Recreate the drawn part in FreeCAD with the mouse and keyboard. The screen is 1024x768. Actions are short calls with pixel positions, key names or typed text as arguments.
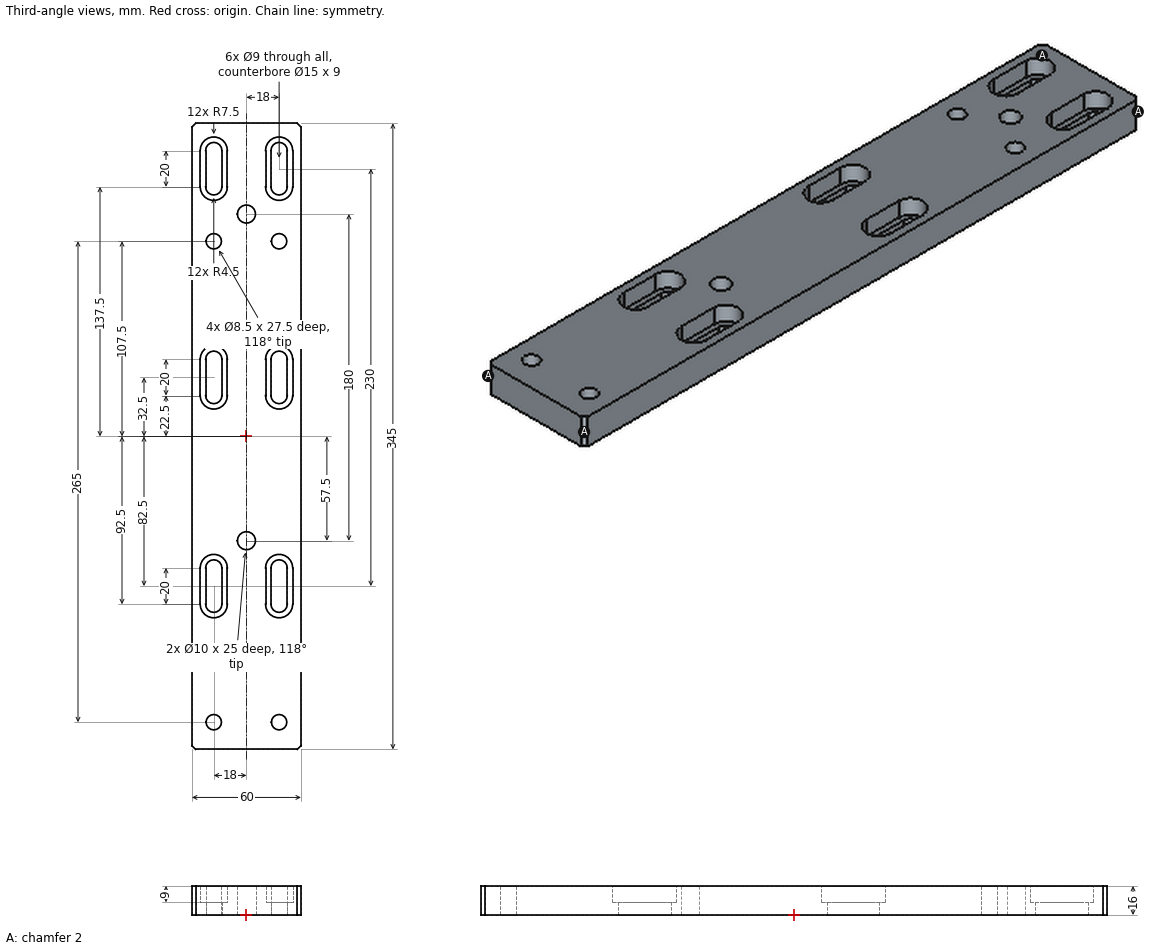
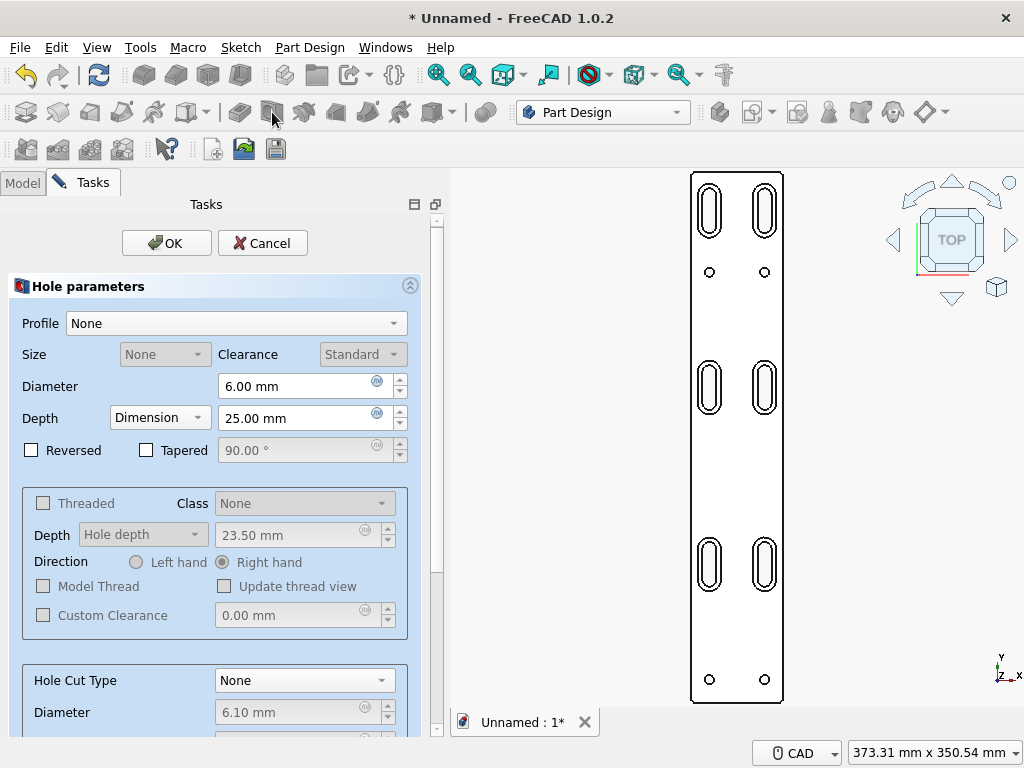
triple_click(305, 386)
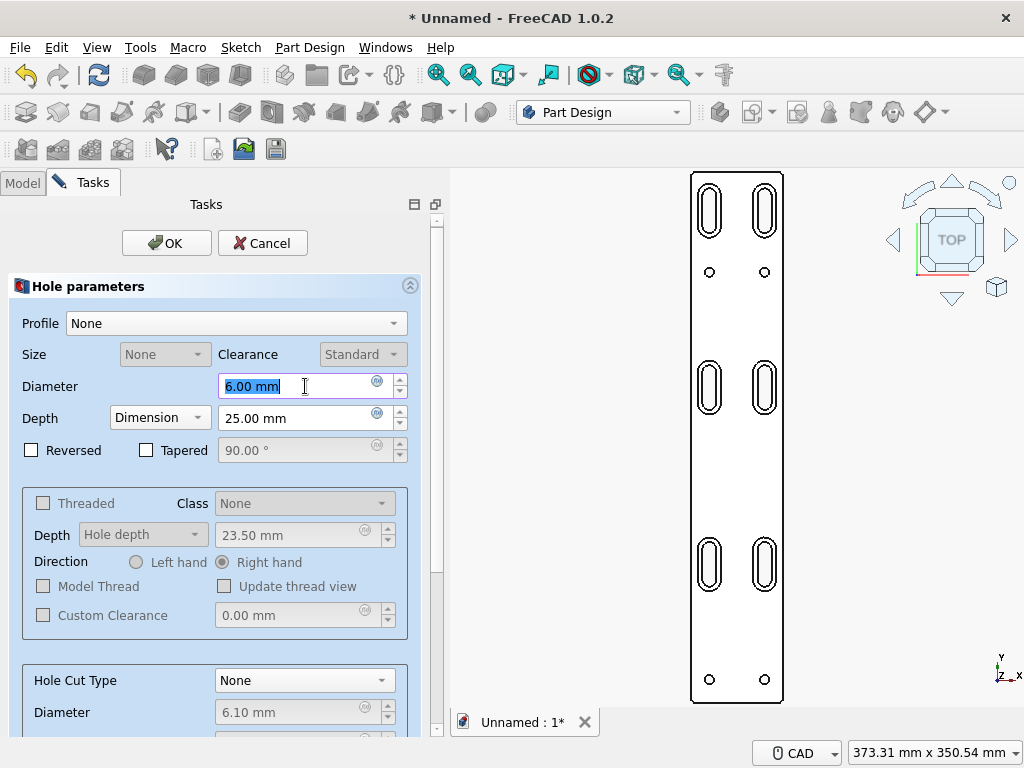
text(8.5)
key(Tab)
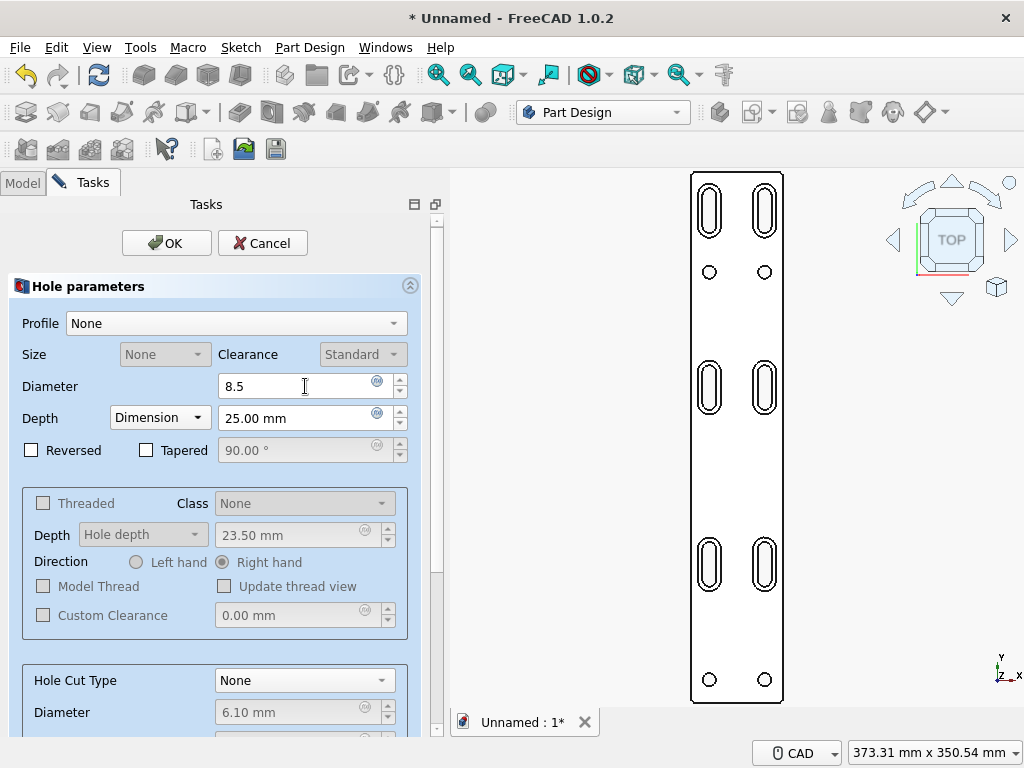
triple_click(305, 418)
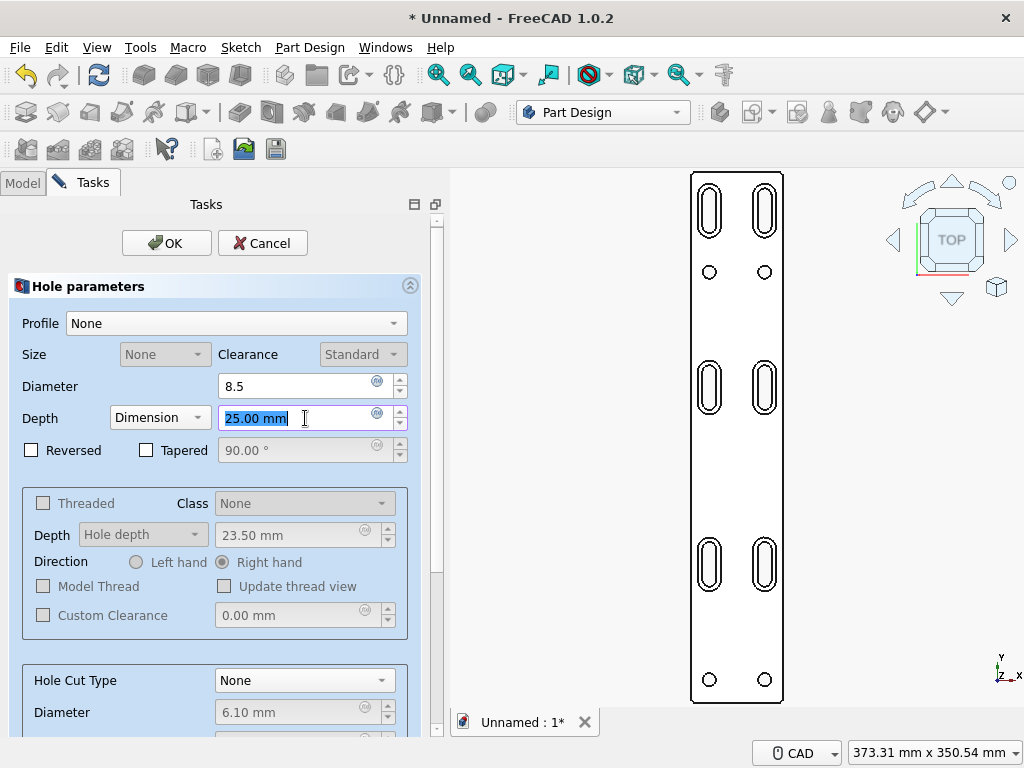
text(27.5)
key(Tab)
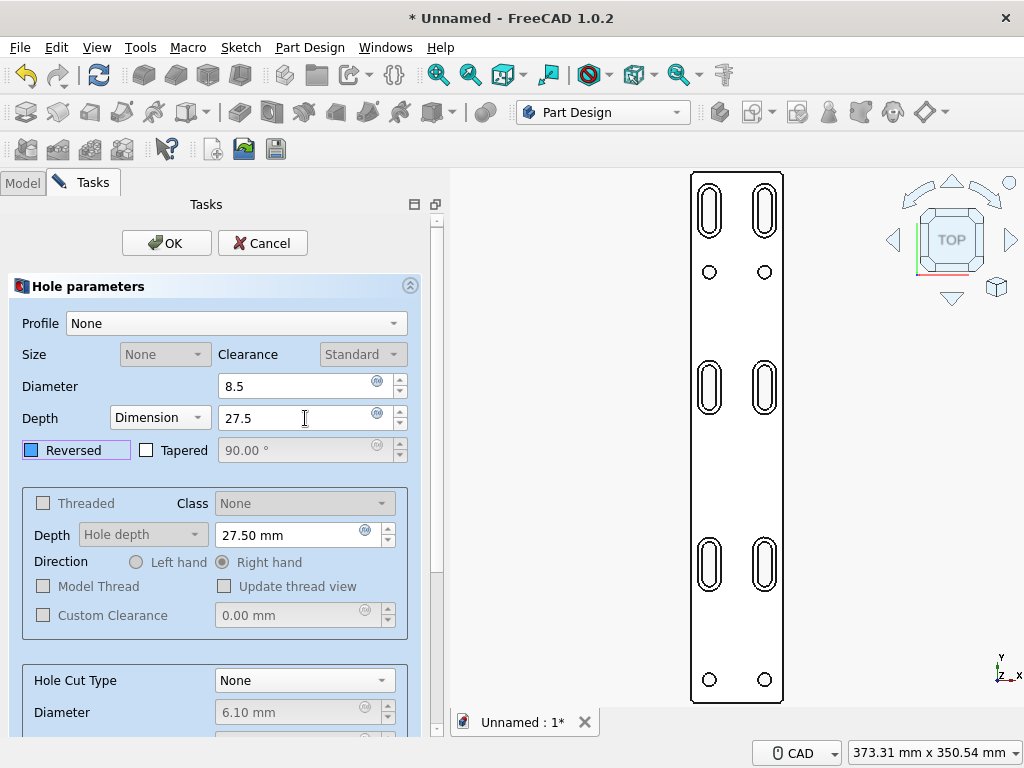
click(167, 243)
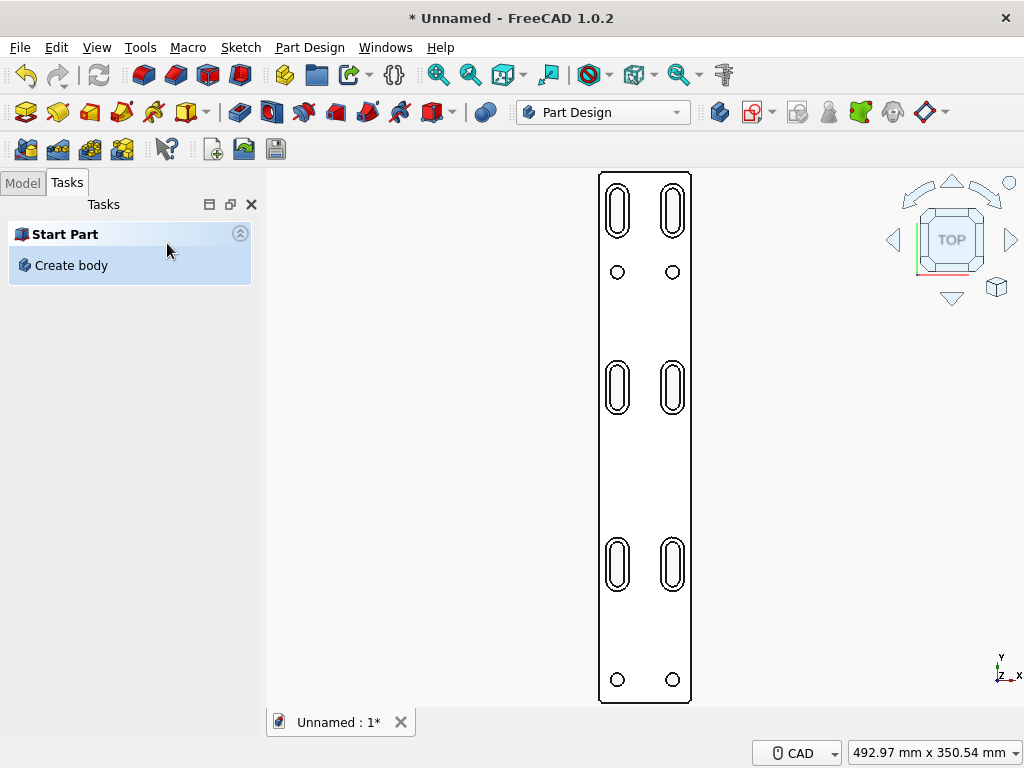
click(645, 512)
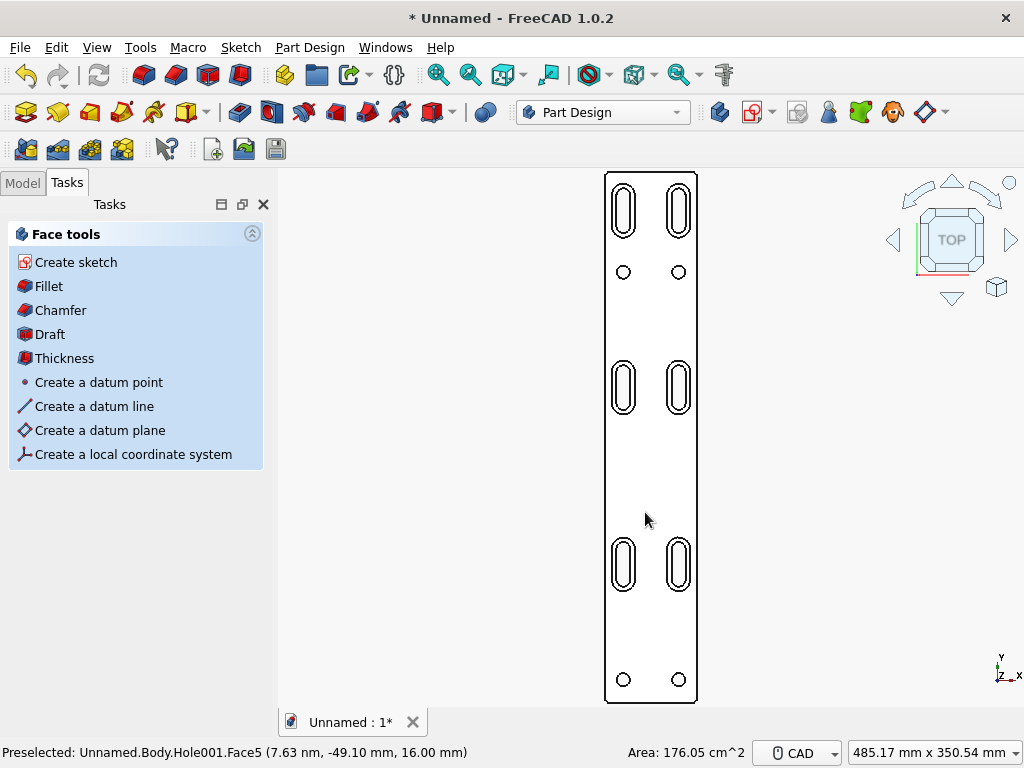
click(752, 112)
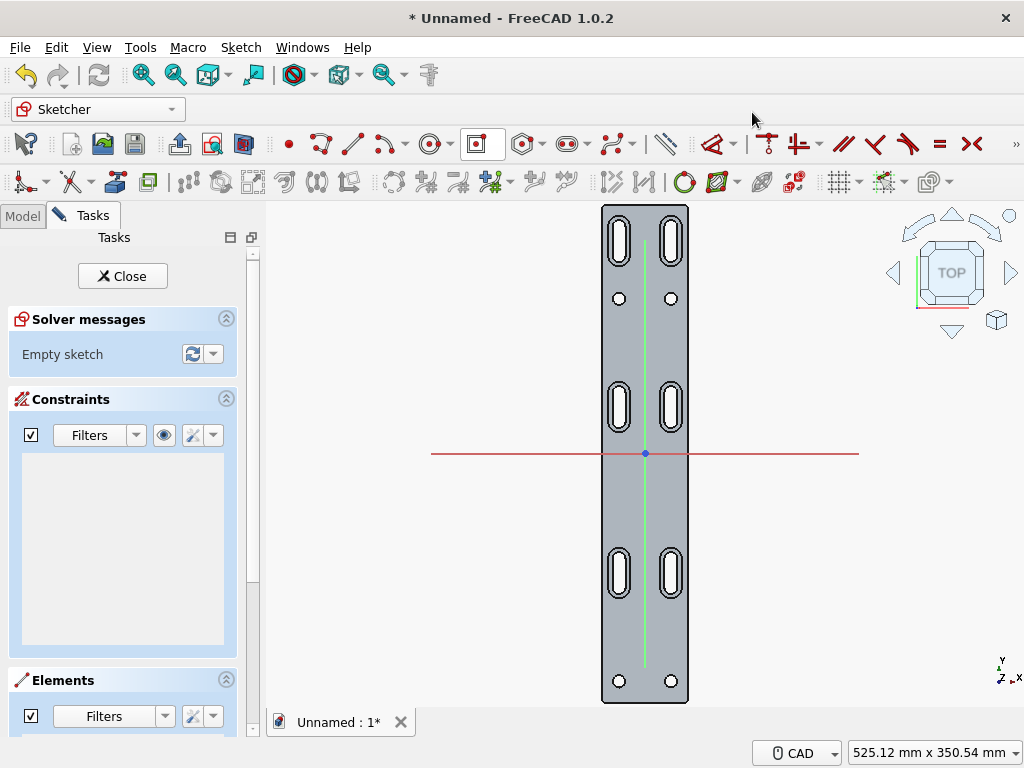
key(g)
key(c)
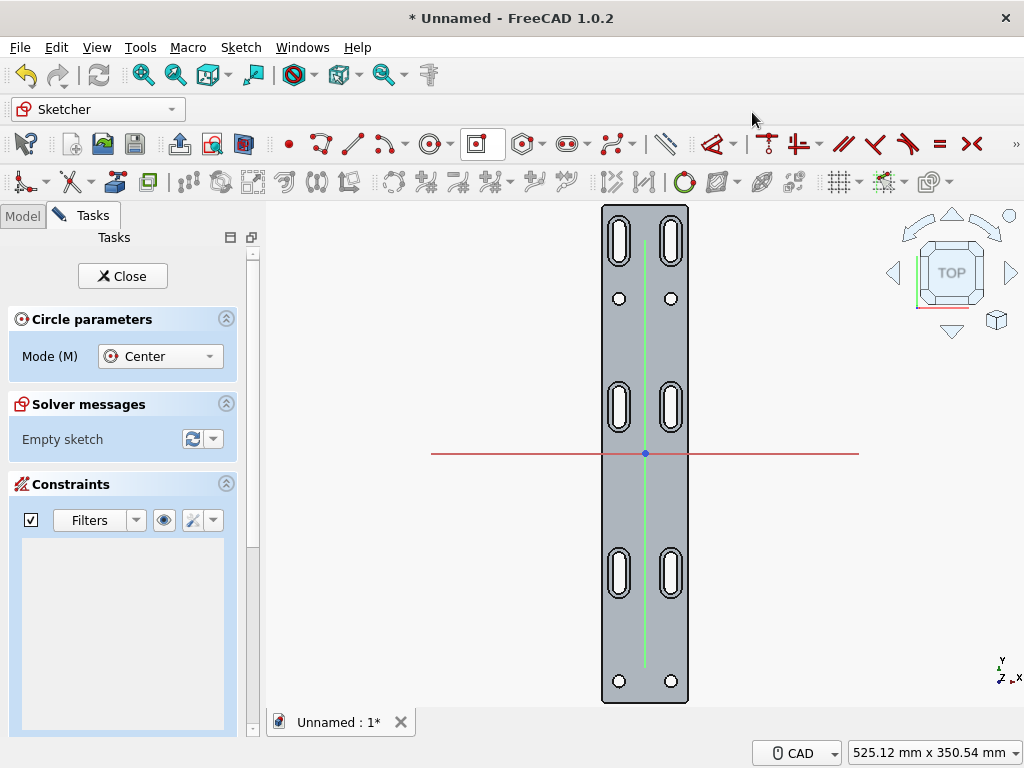
scroll(645, 537, up, 6)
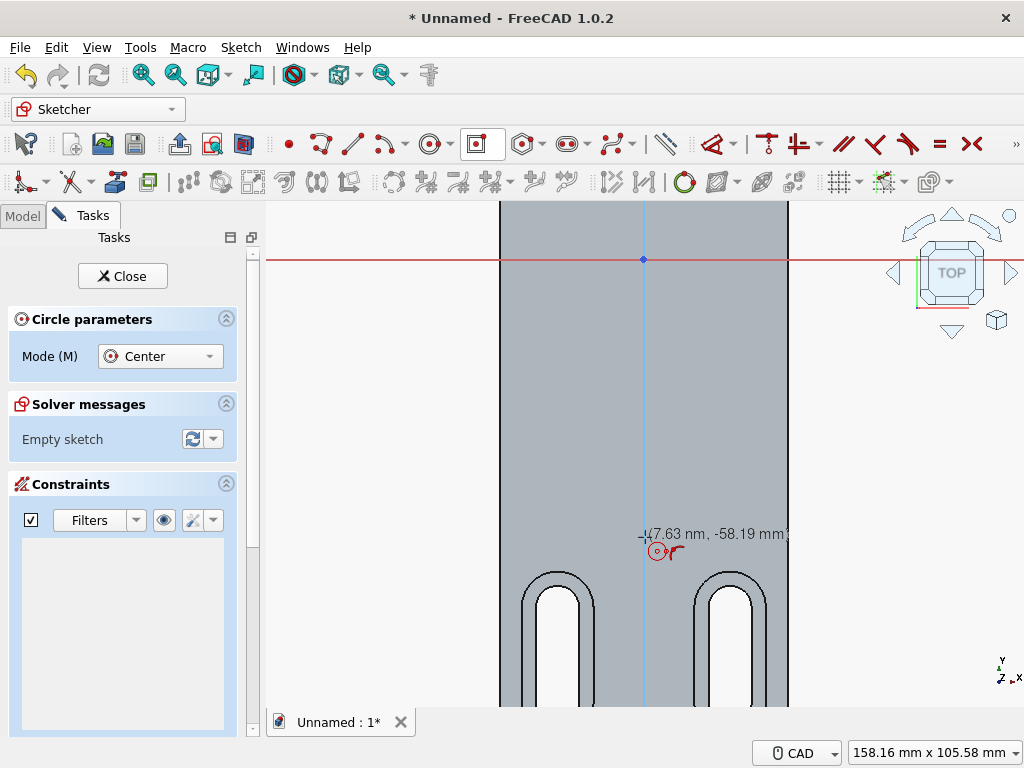
click(644, 535)
click(661, 519)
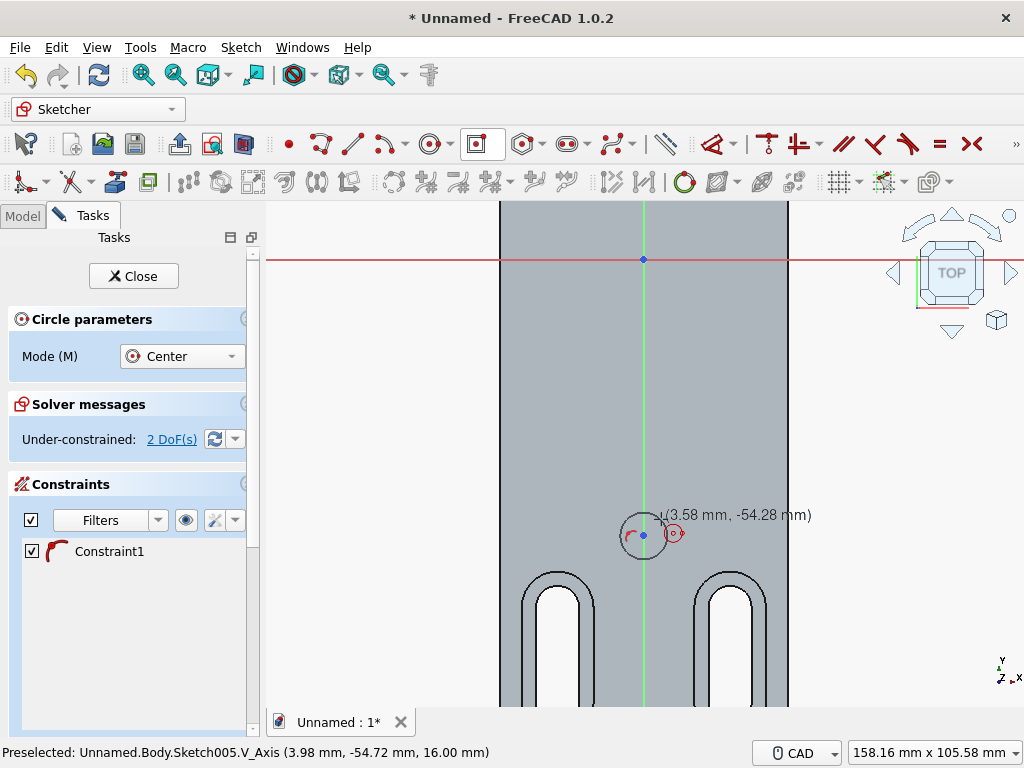
scroll(537, 658, down, 5)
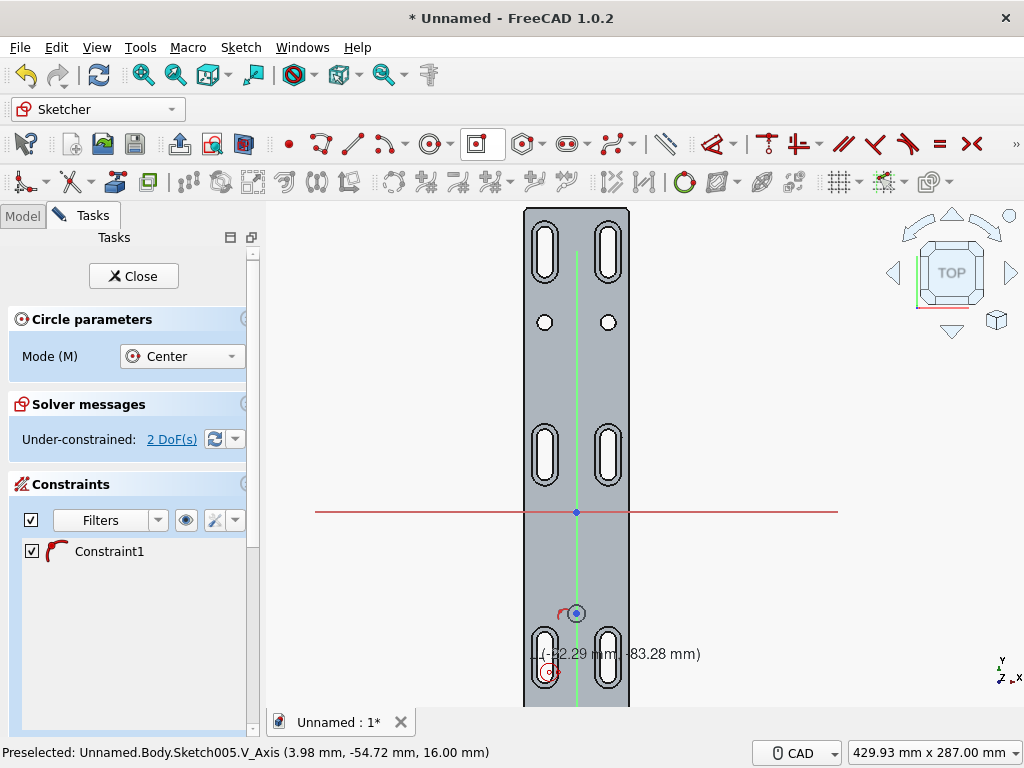
scroll(577, 296, up, 5)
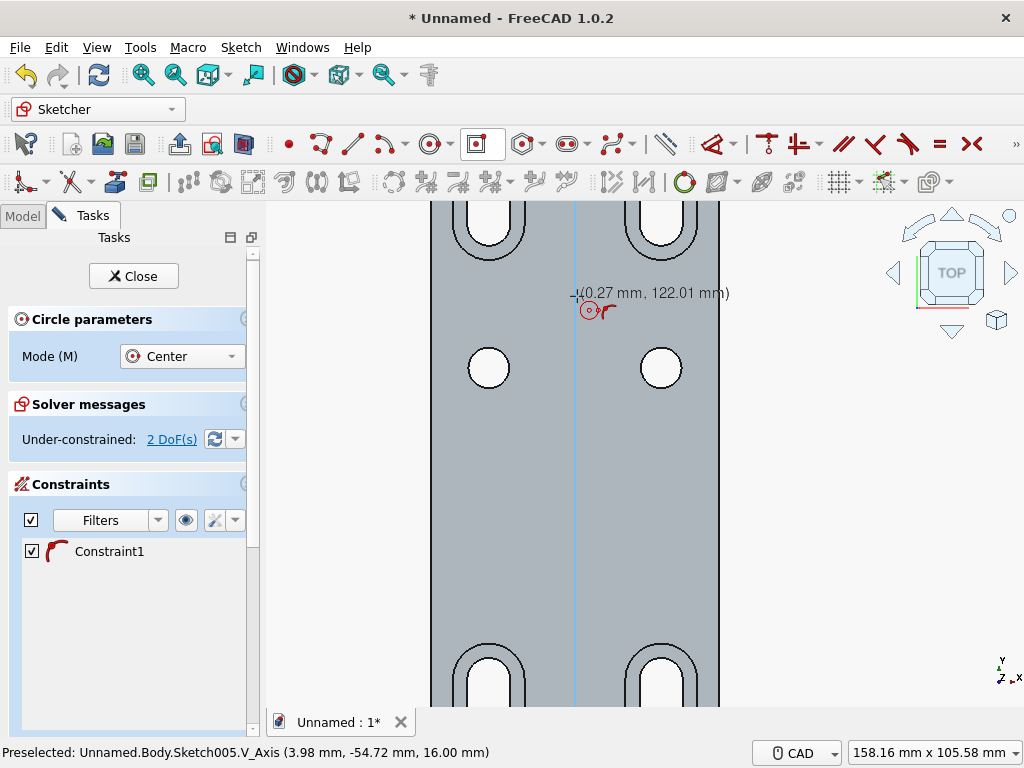
click(575, 296)
click(592, 279)
key(Escape)